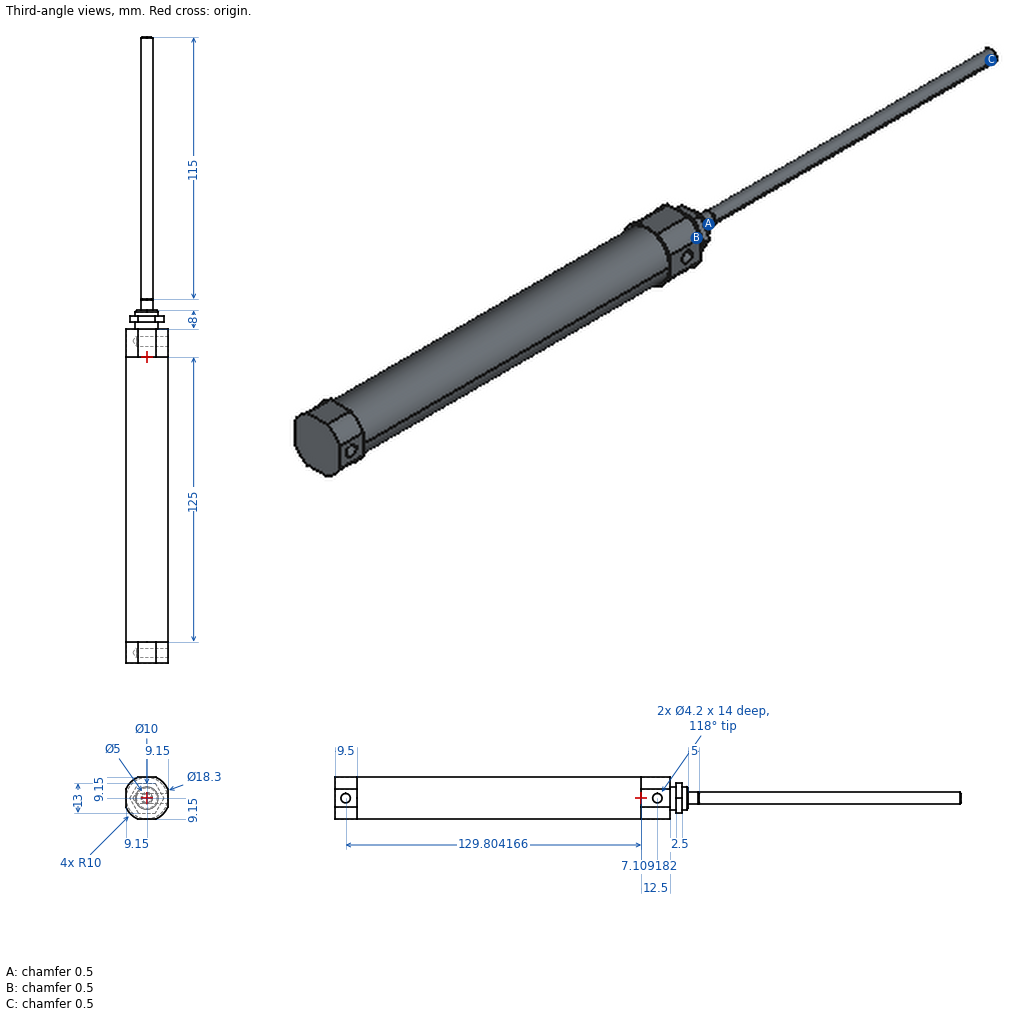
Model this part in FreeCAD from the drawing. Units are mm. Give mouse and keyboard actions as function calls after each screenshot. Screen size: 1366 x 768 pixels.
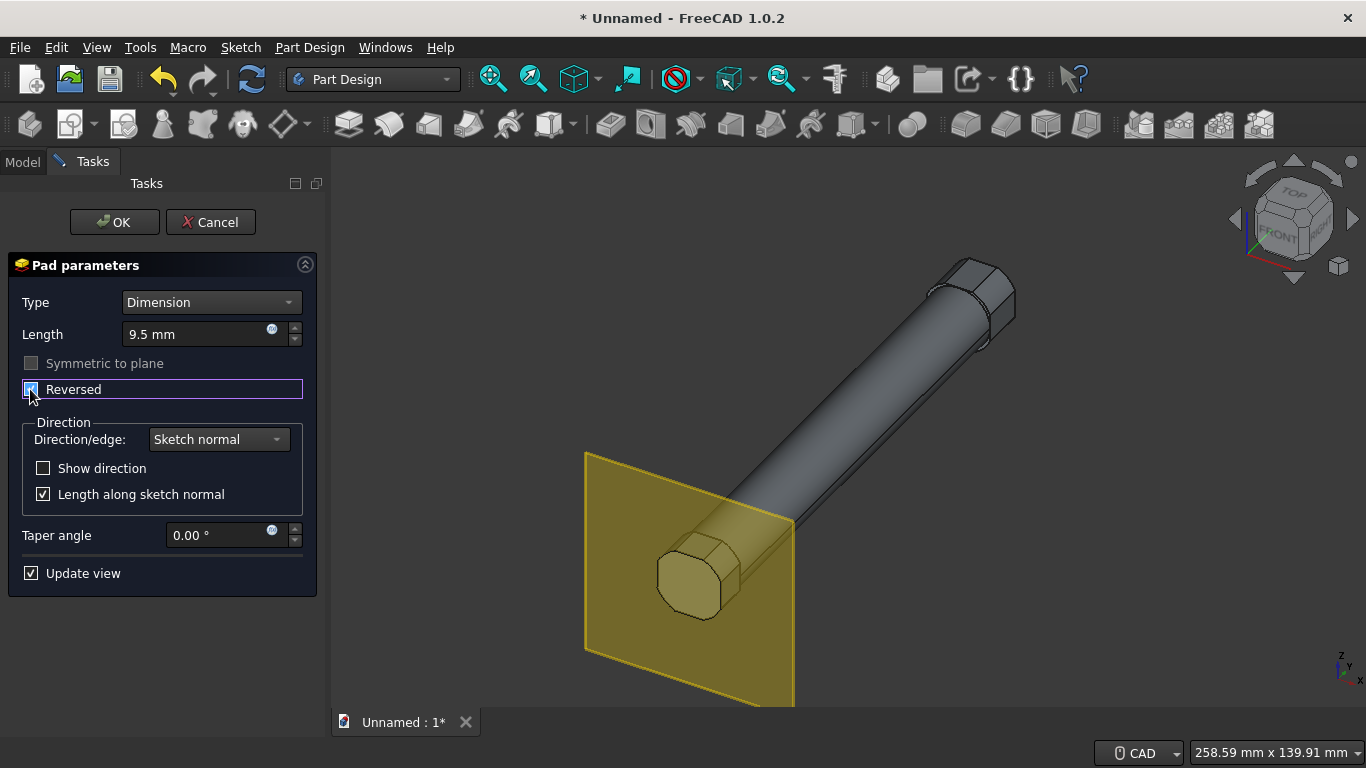
click(115, 222)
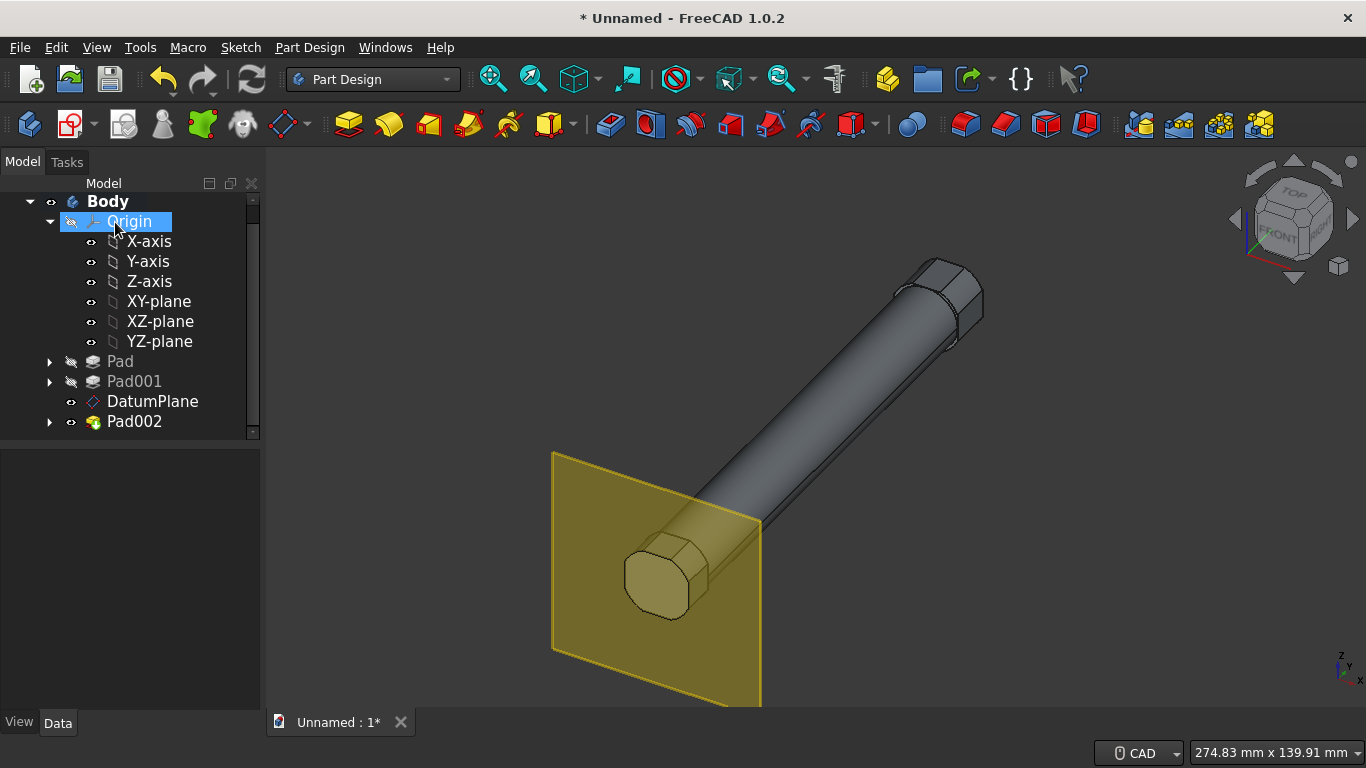
click(116, 402)
key(space)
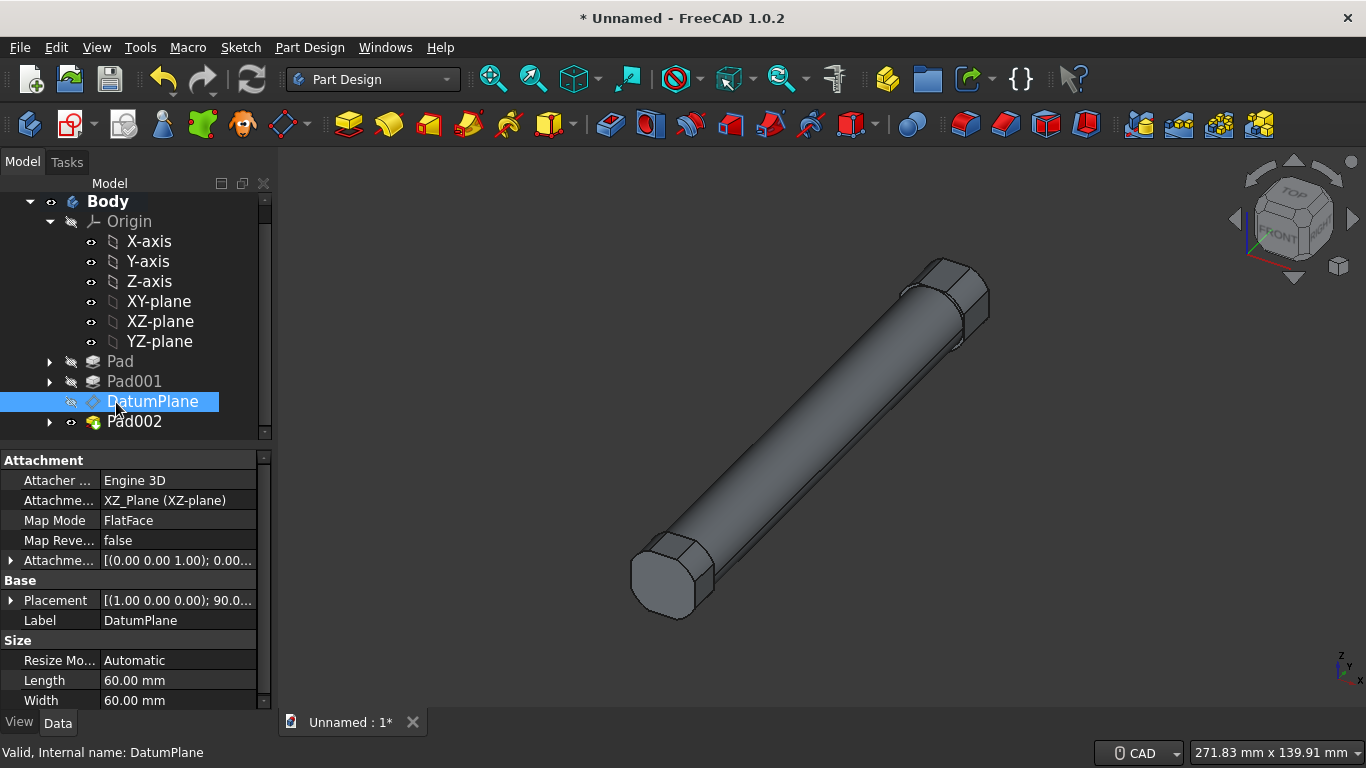
key(4)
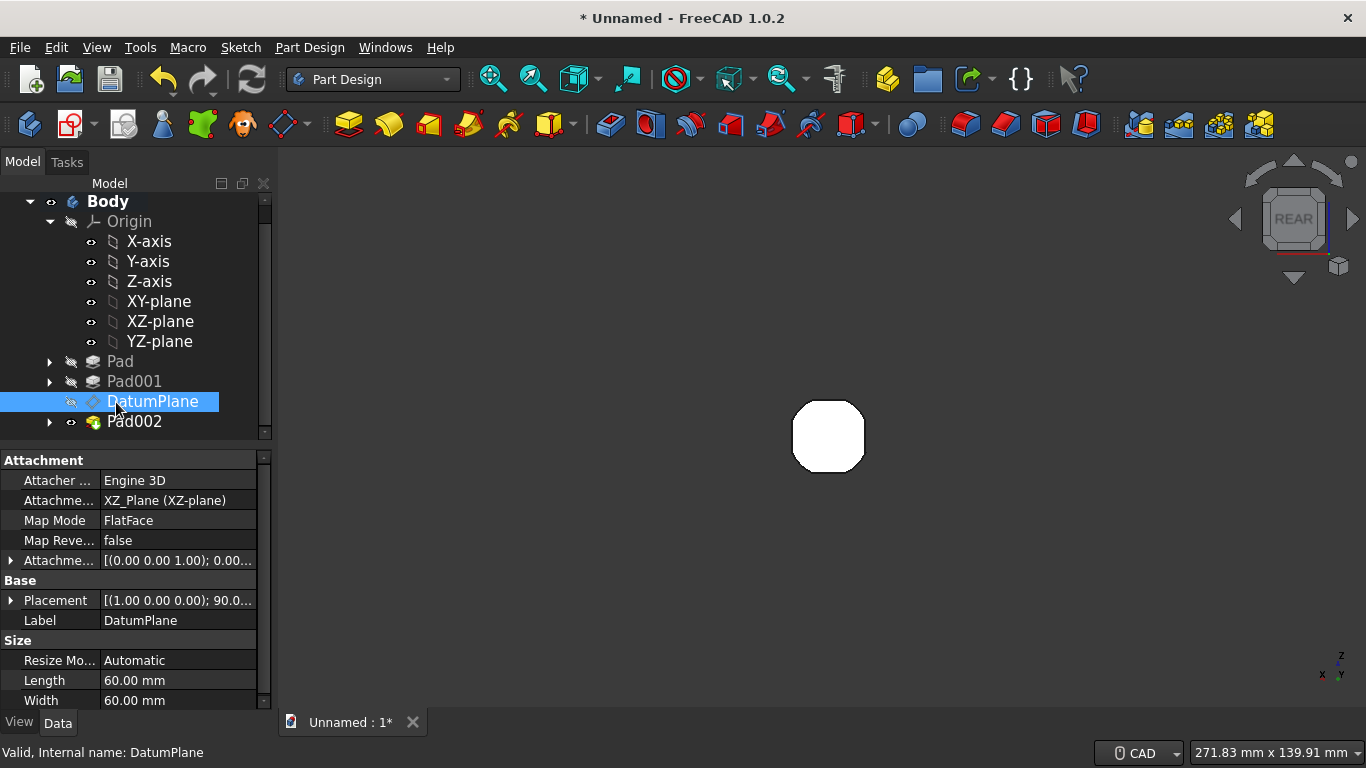
key(v)
key(f)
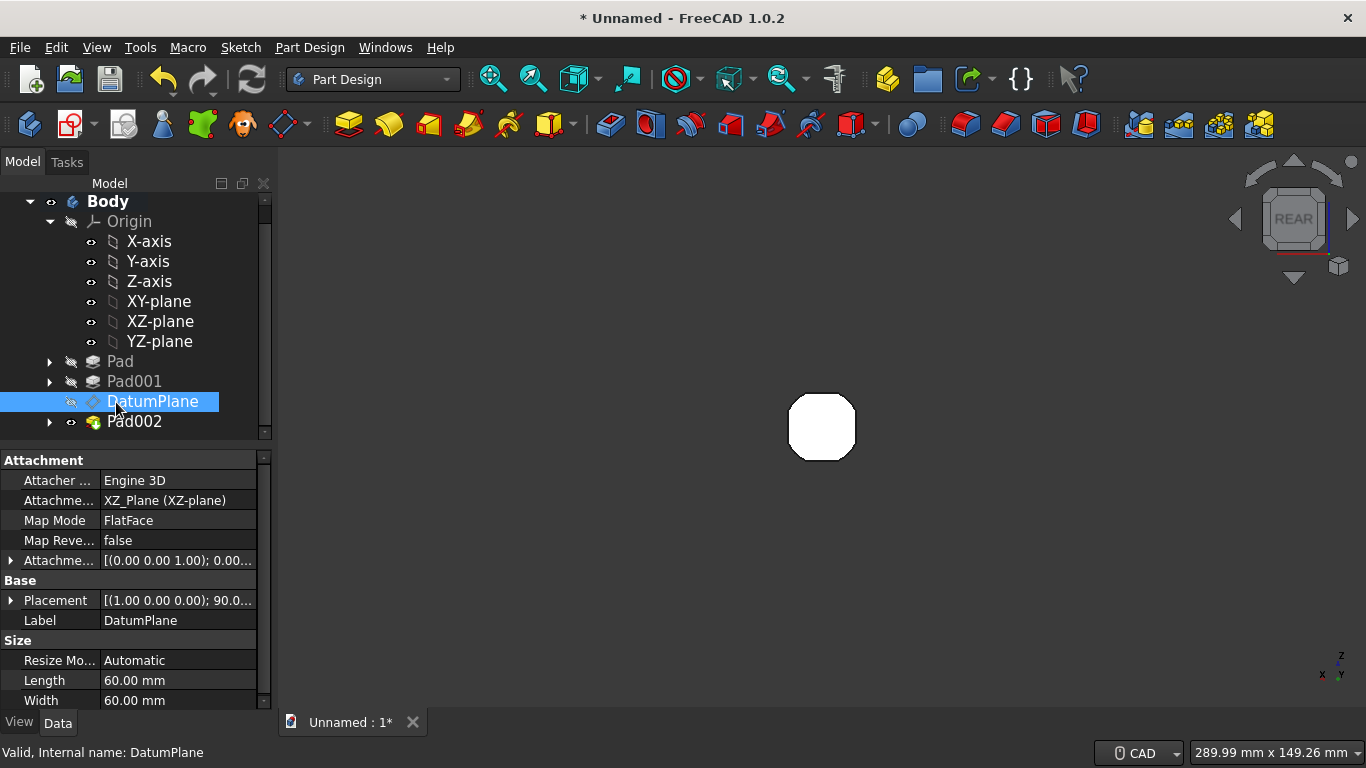
click(822, 426)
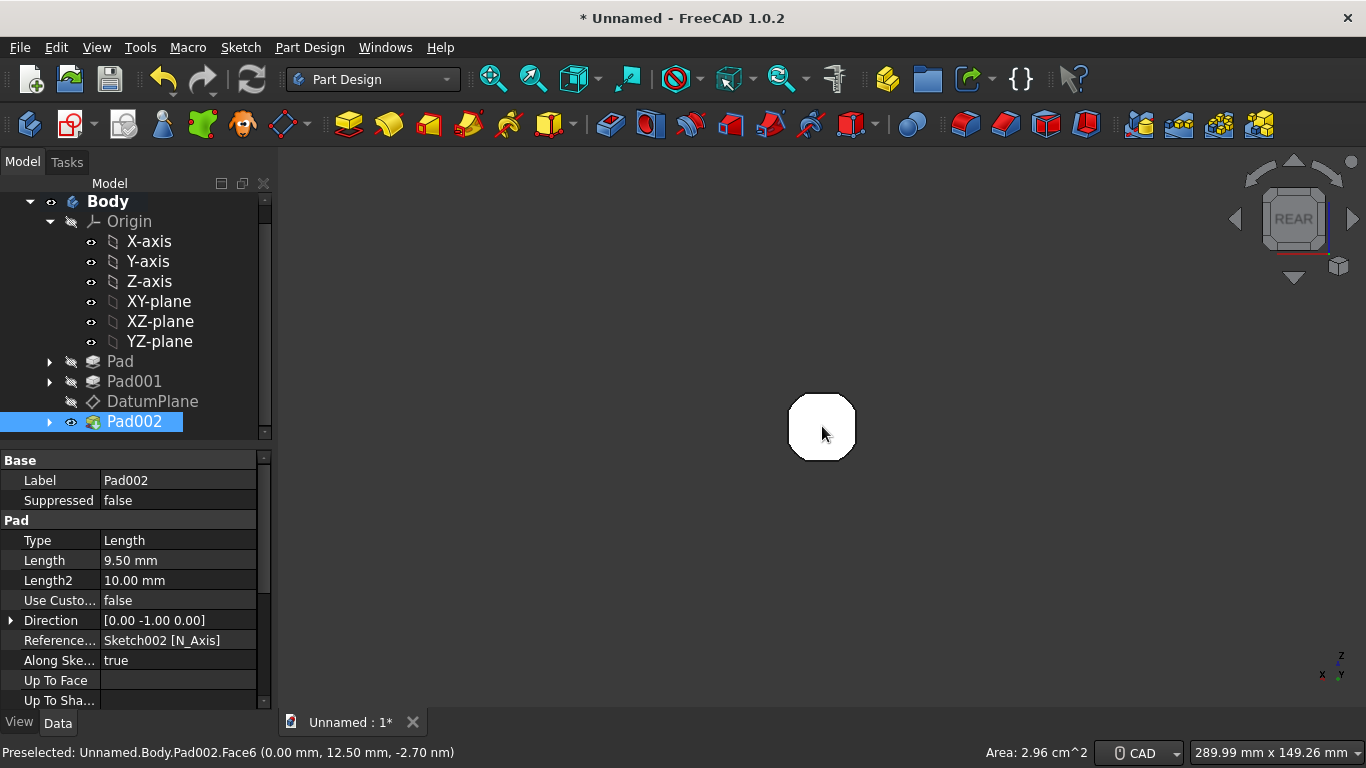
click(70, 124)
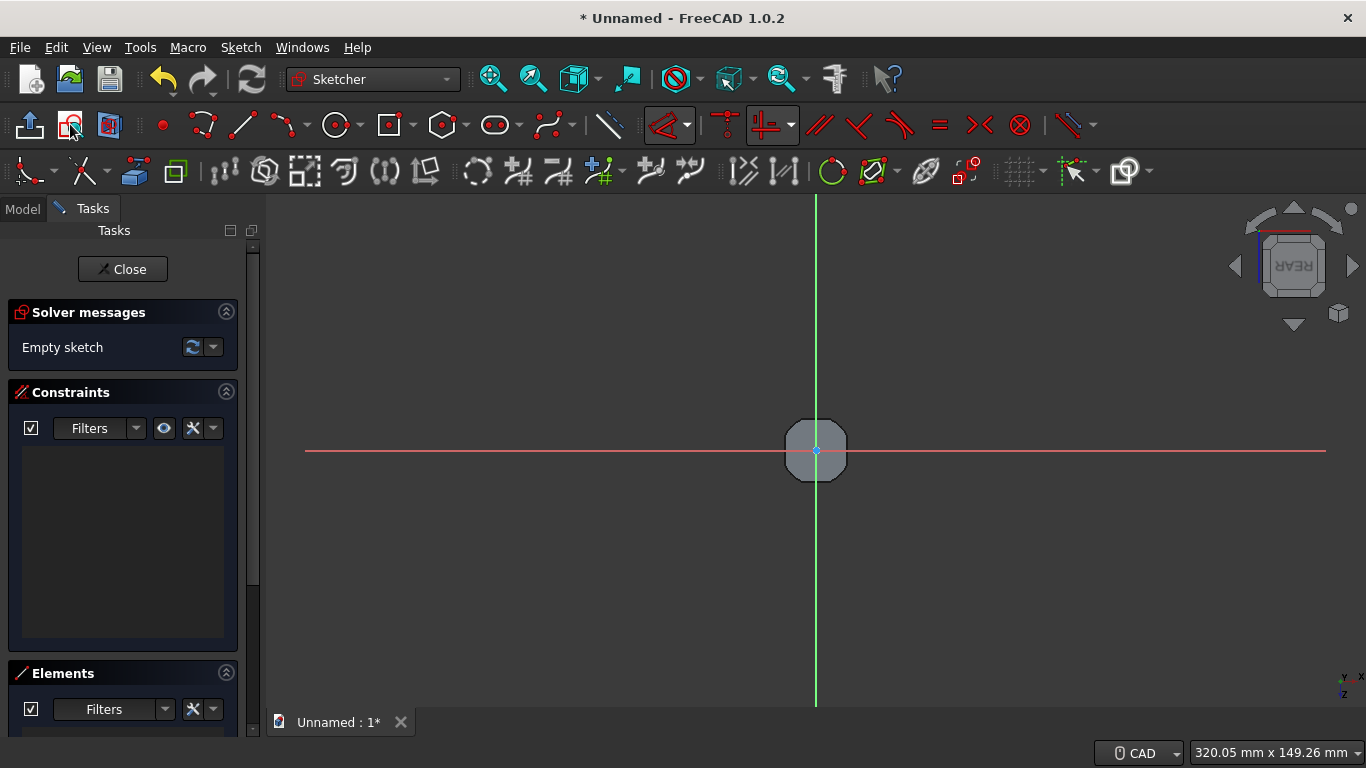
scroll(825, 451, up, 11)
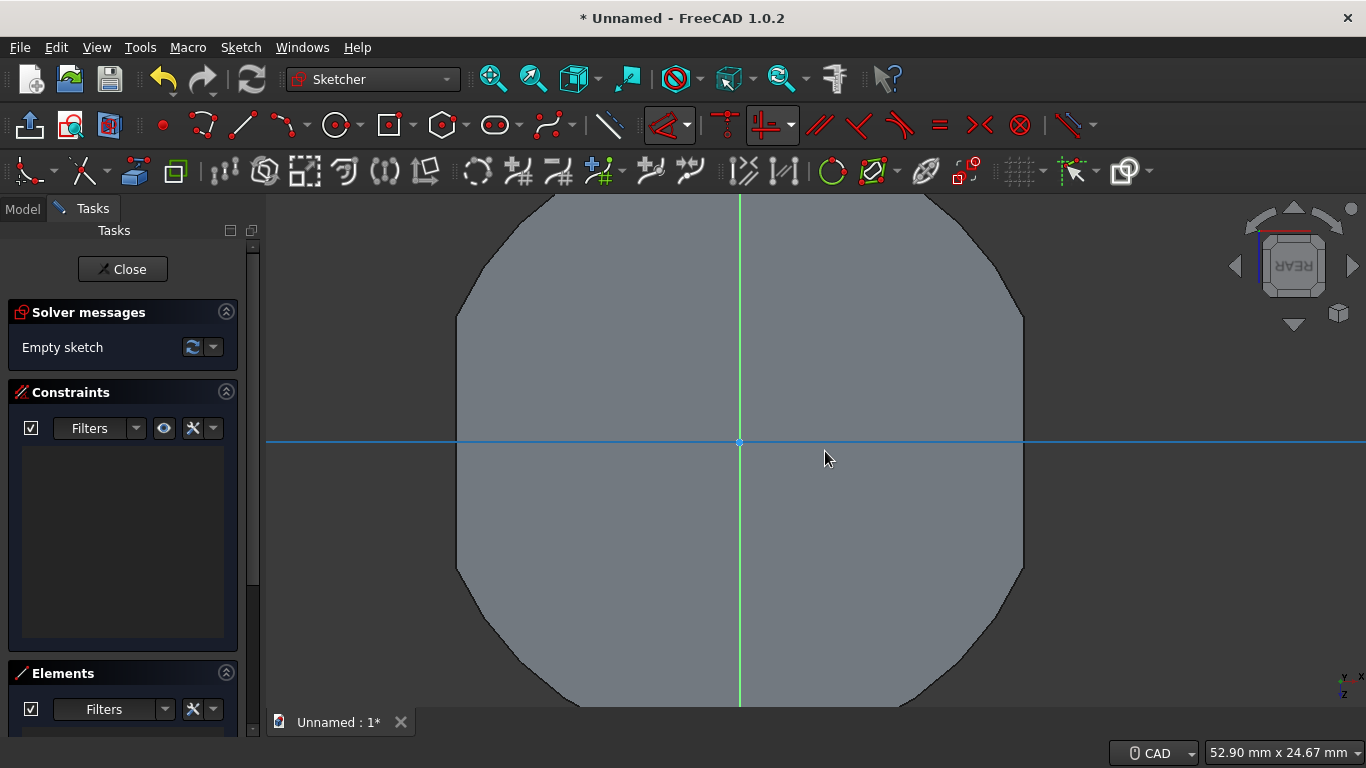
click(336, 126)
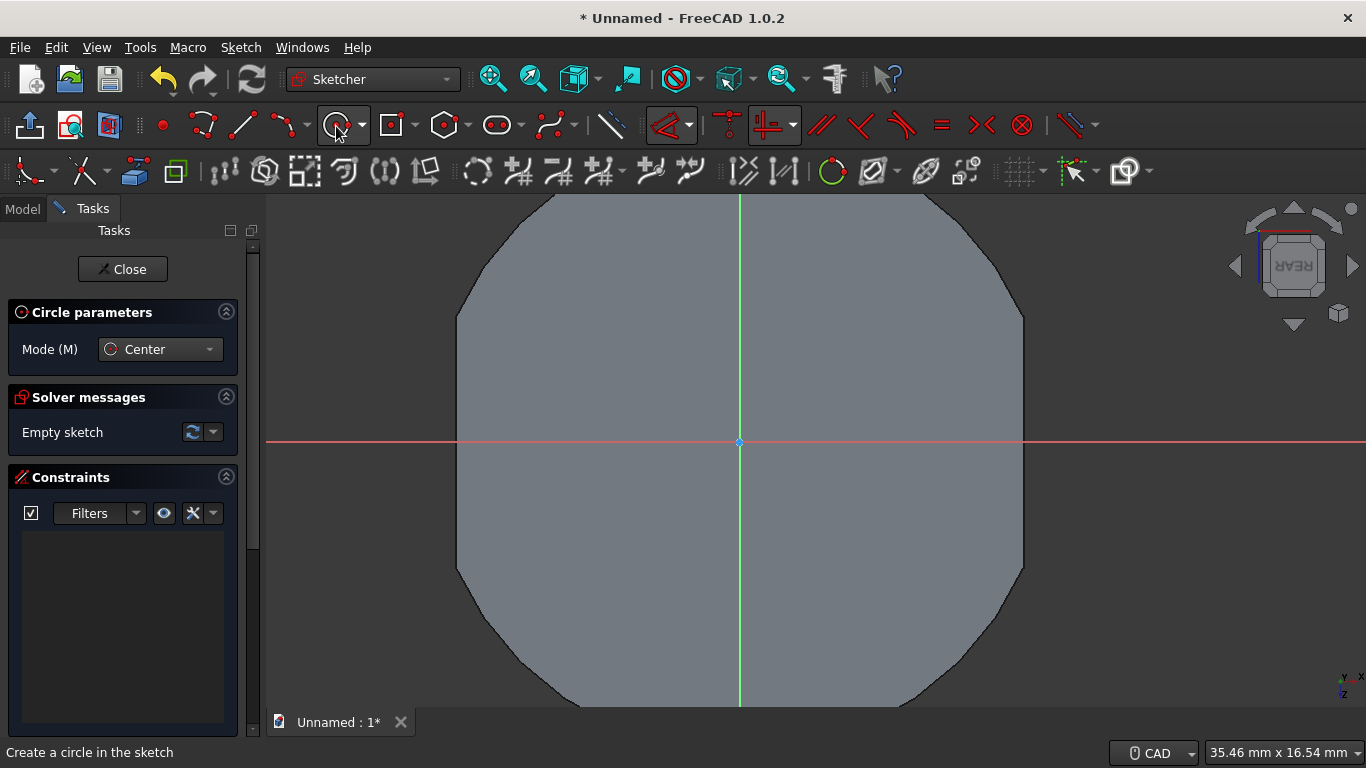
click(740, 442)
click(849, 333)
key(Escape)